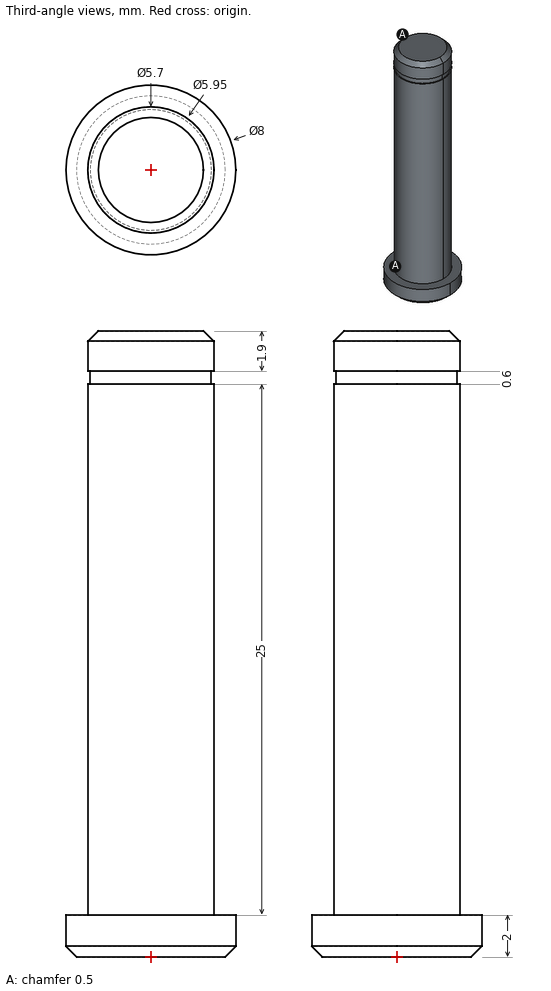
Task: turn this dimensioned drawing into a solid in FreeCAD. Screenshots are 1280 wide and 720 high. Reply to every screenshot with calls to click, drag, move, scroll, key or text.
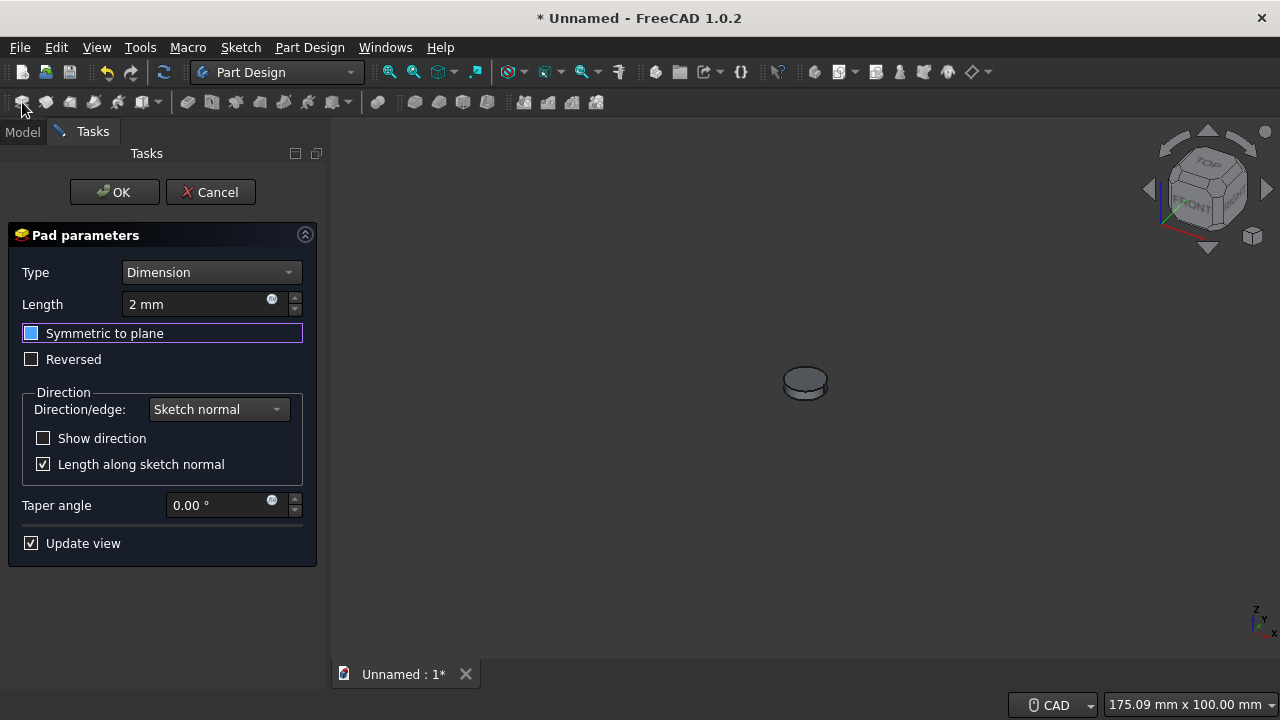
click(115, 192)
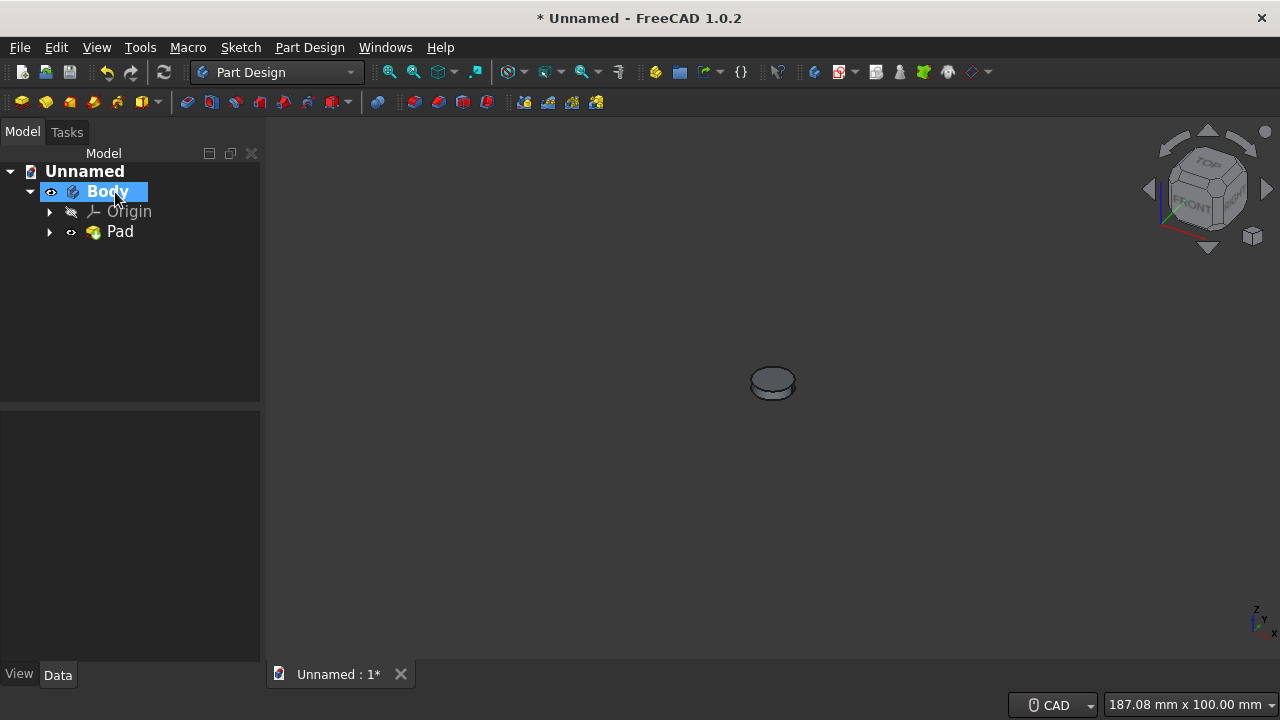
key(v)
key(f)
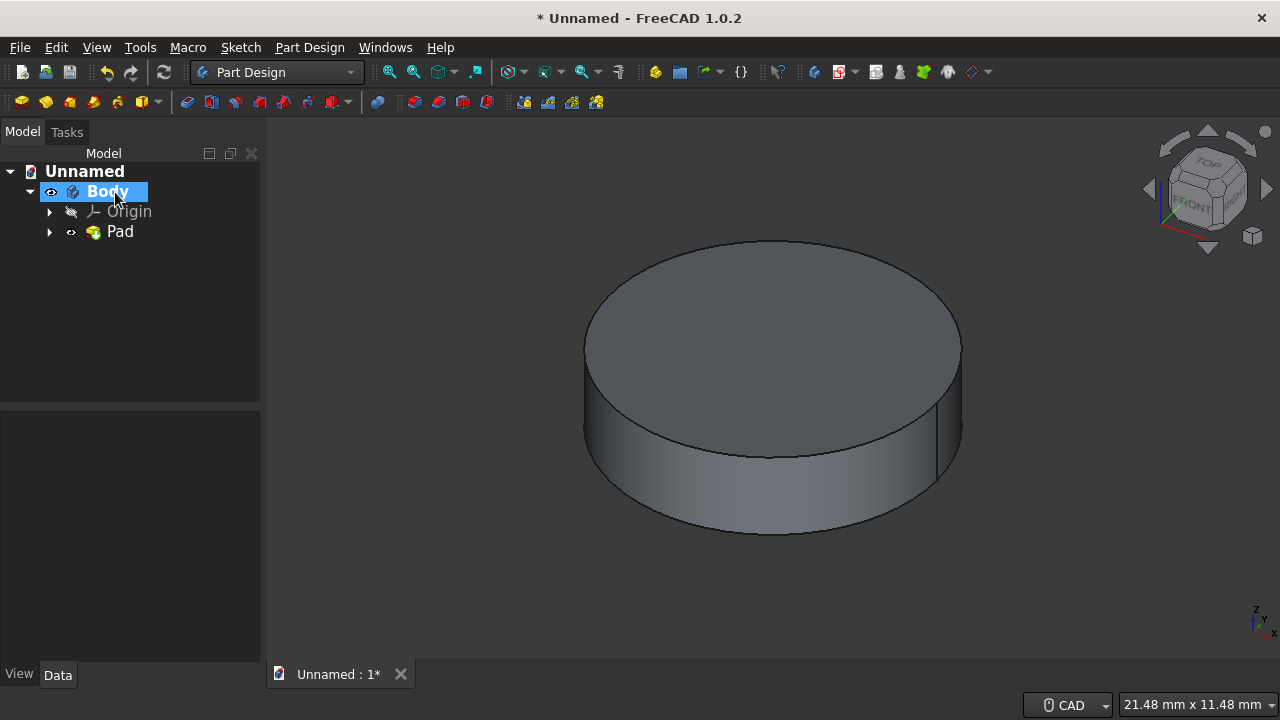
click(773, 348)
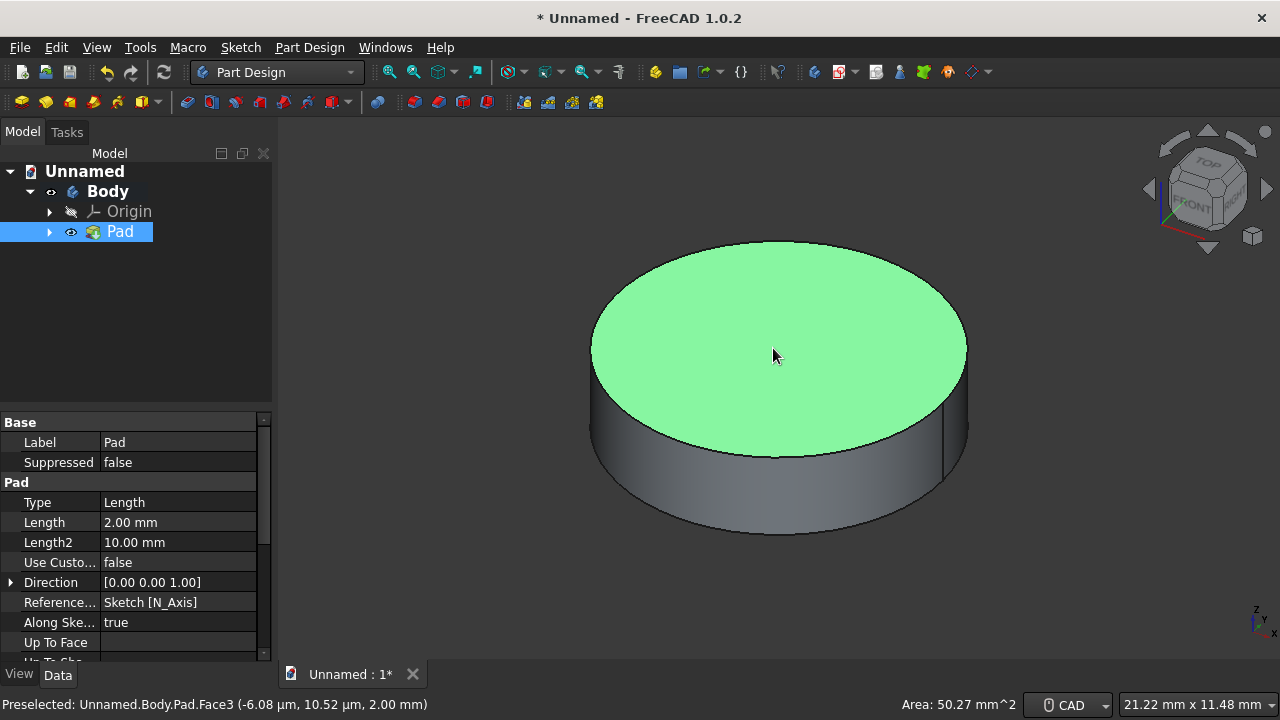
click(840, 72)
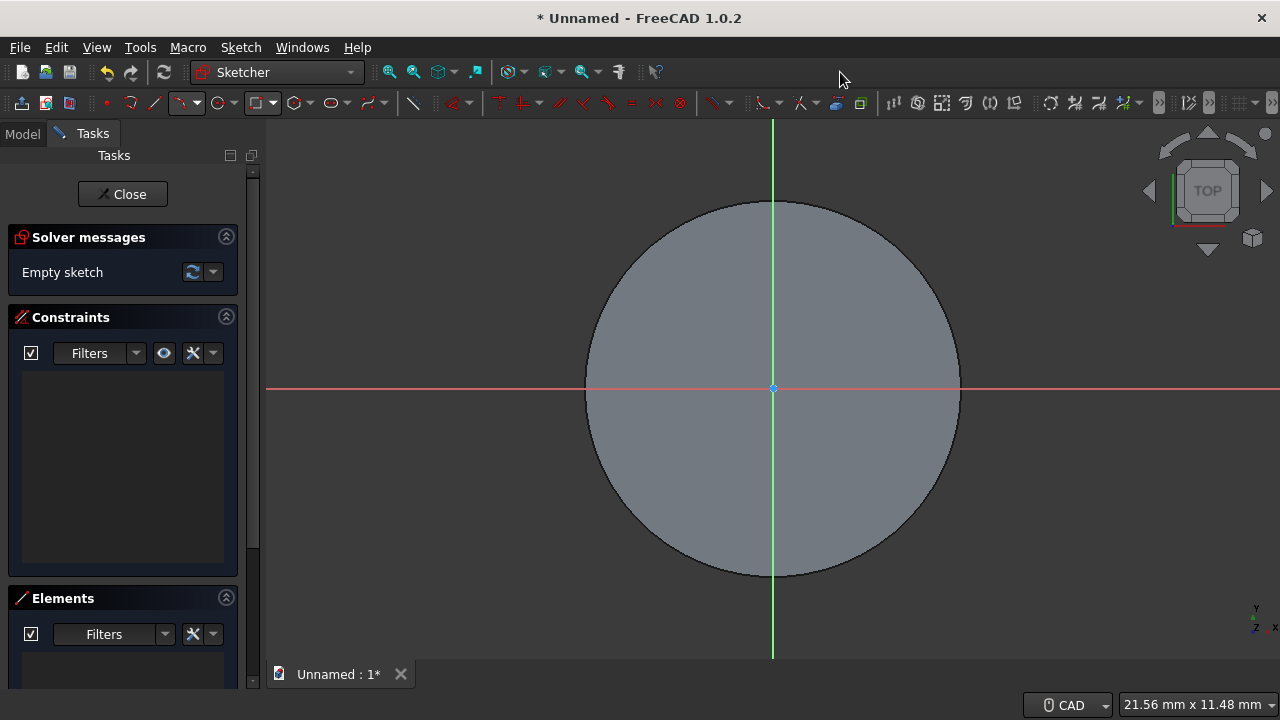
click(218, 104)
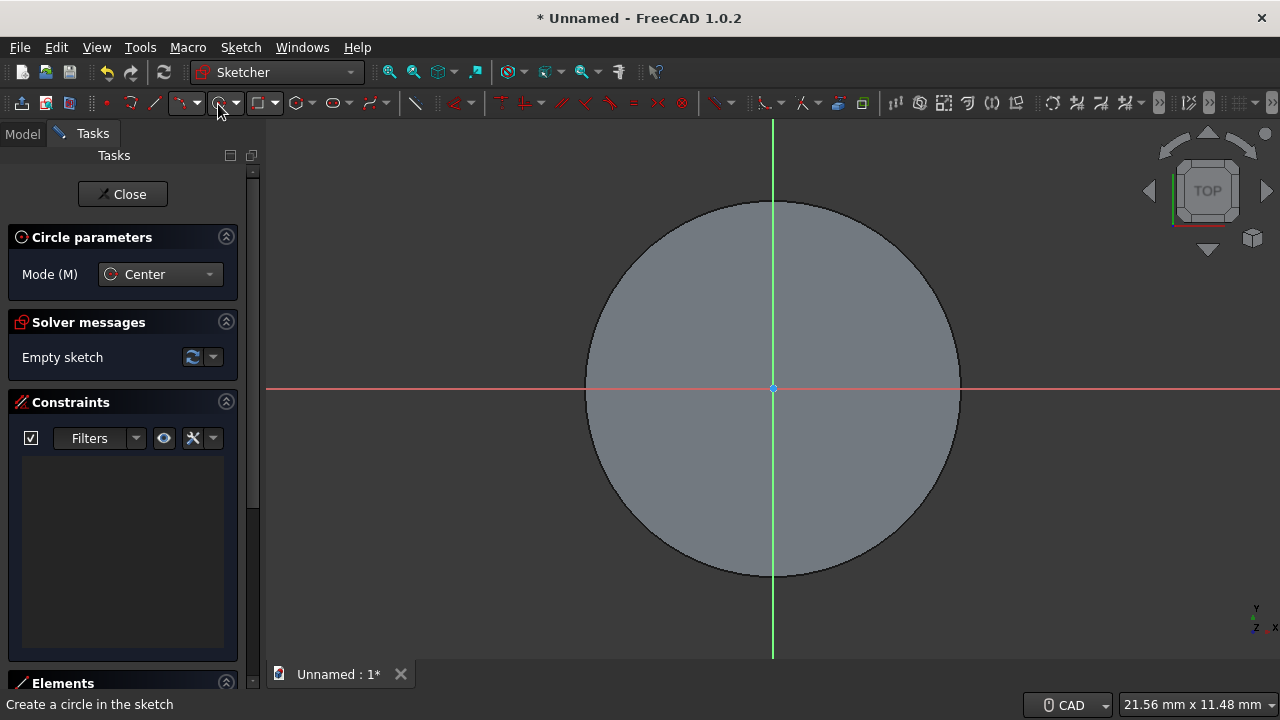
click(773, 389)
move(872, 290)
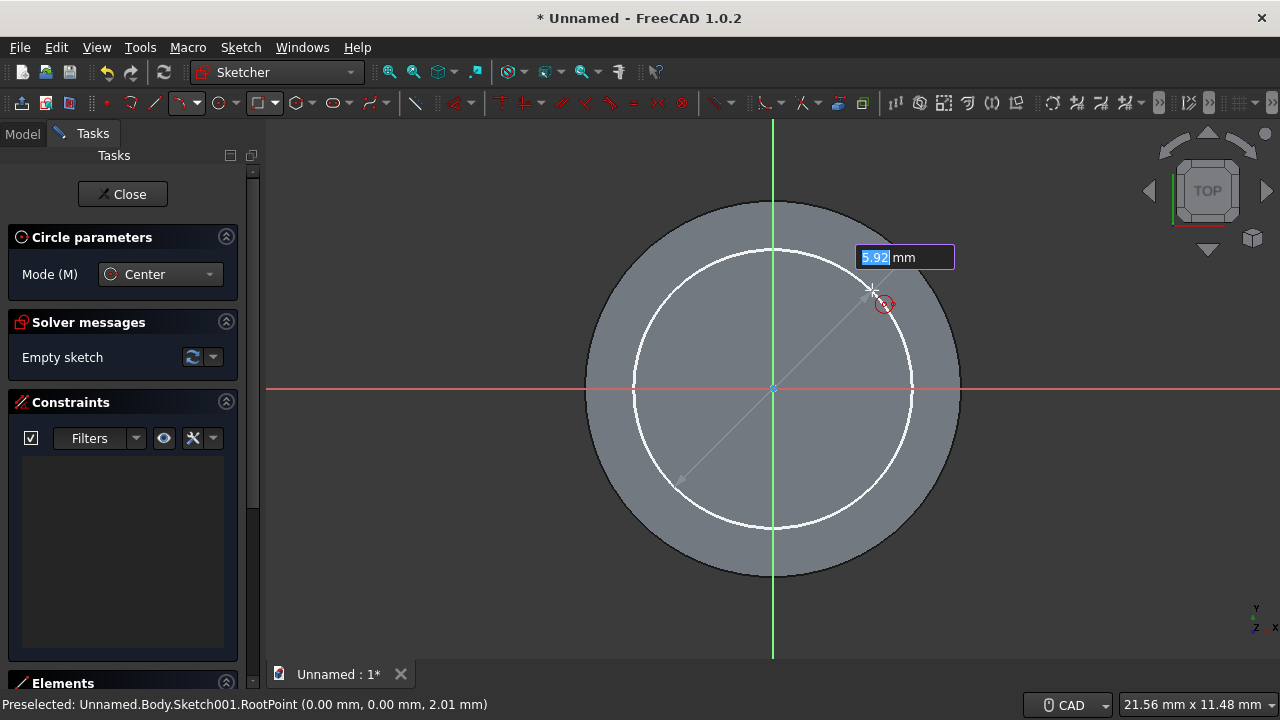
text(5.95)
key(Return)
key(Escape)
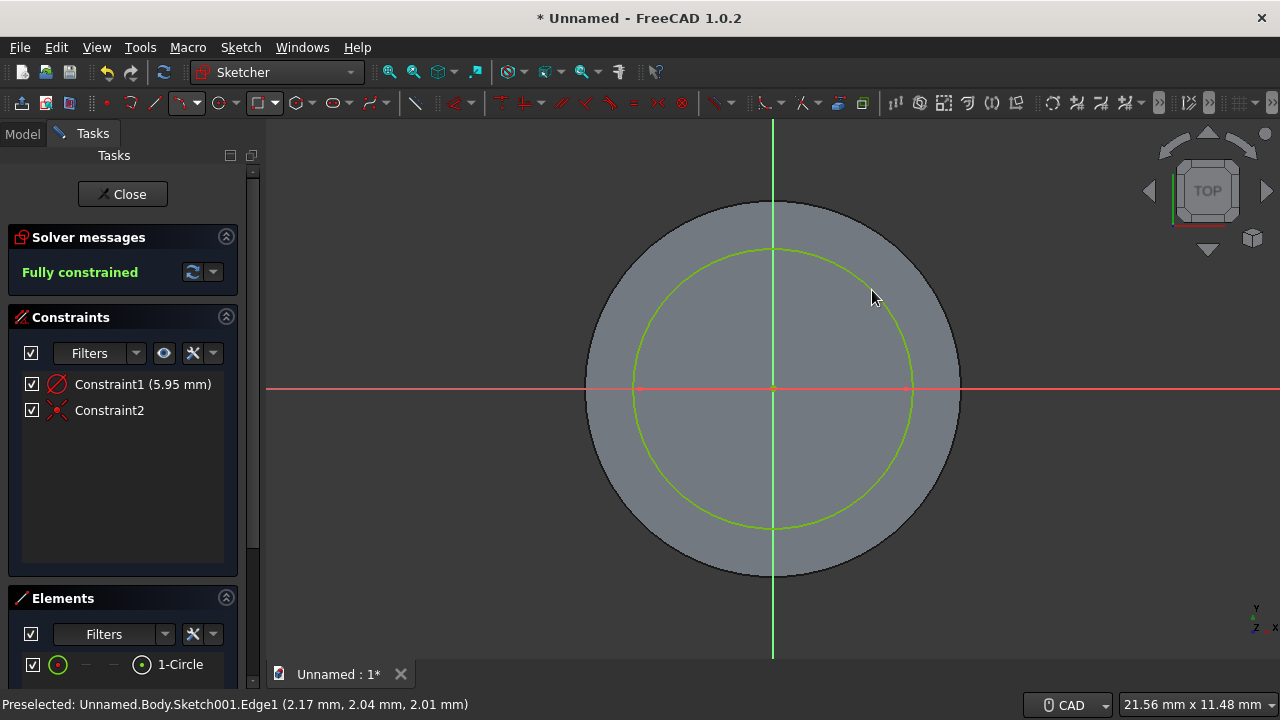
click(123, 194)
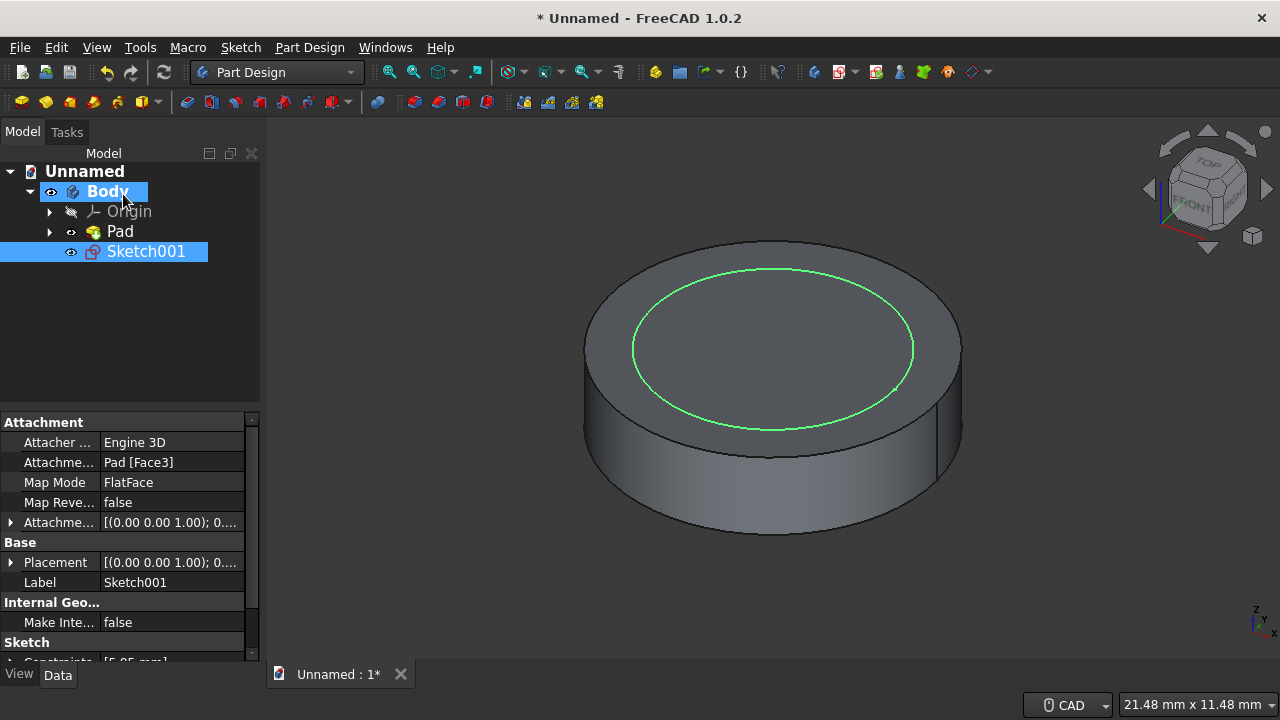
click(22, 102)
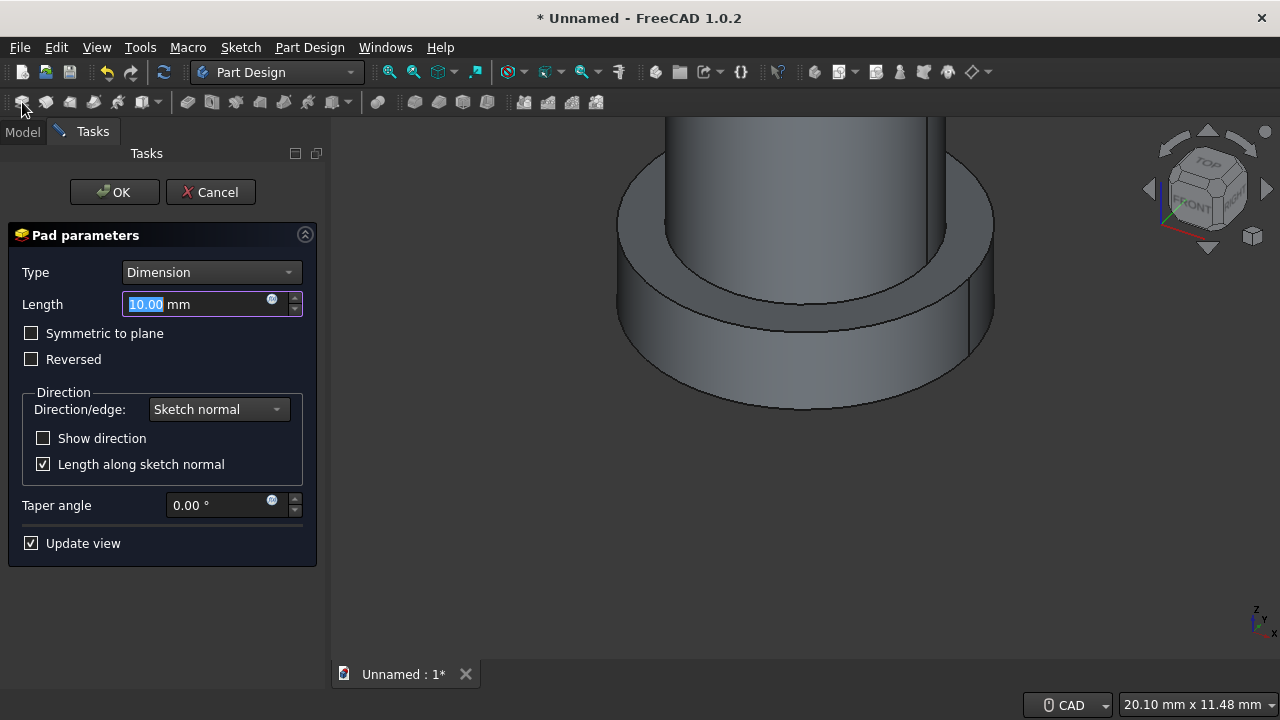
text(25)
key(Tab)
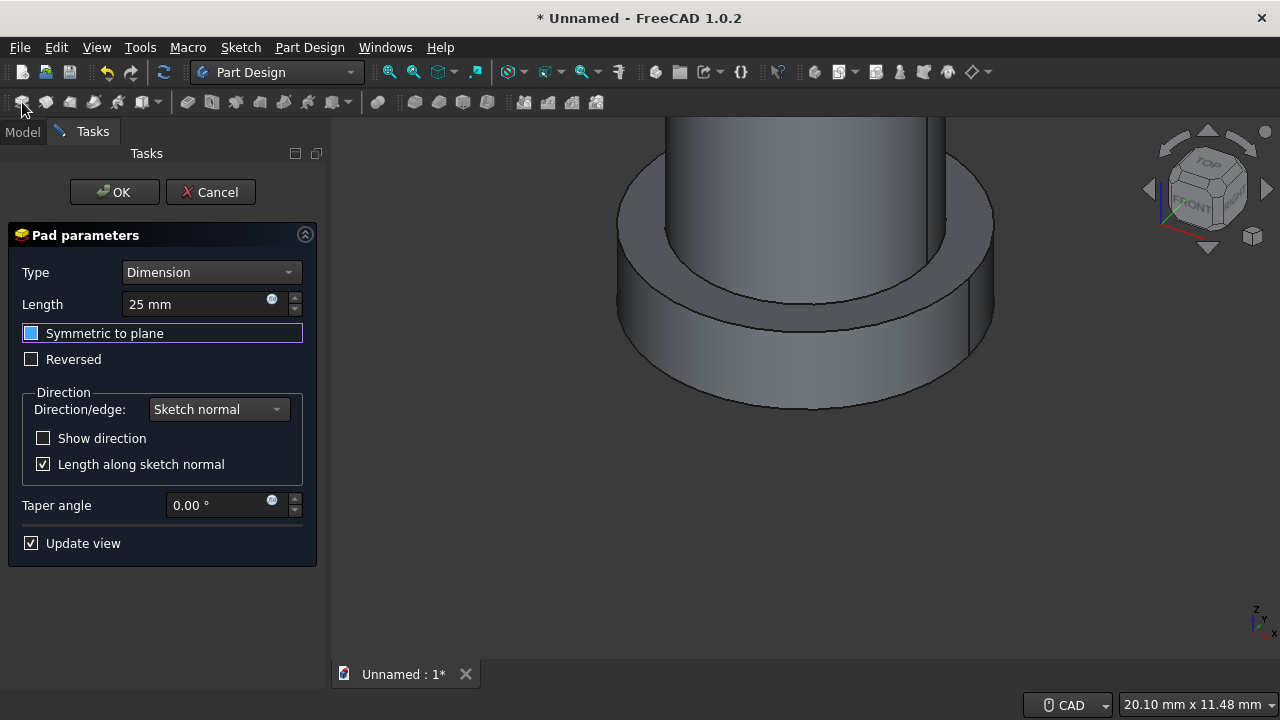
click(115, 192)